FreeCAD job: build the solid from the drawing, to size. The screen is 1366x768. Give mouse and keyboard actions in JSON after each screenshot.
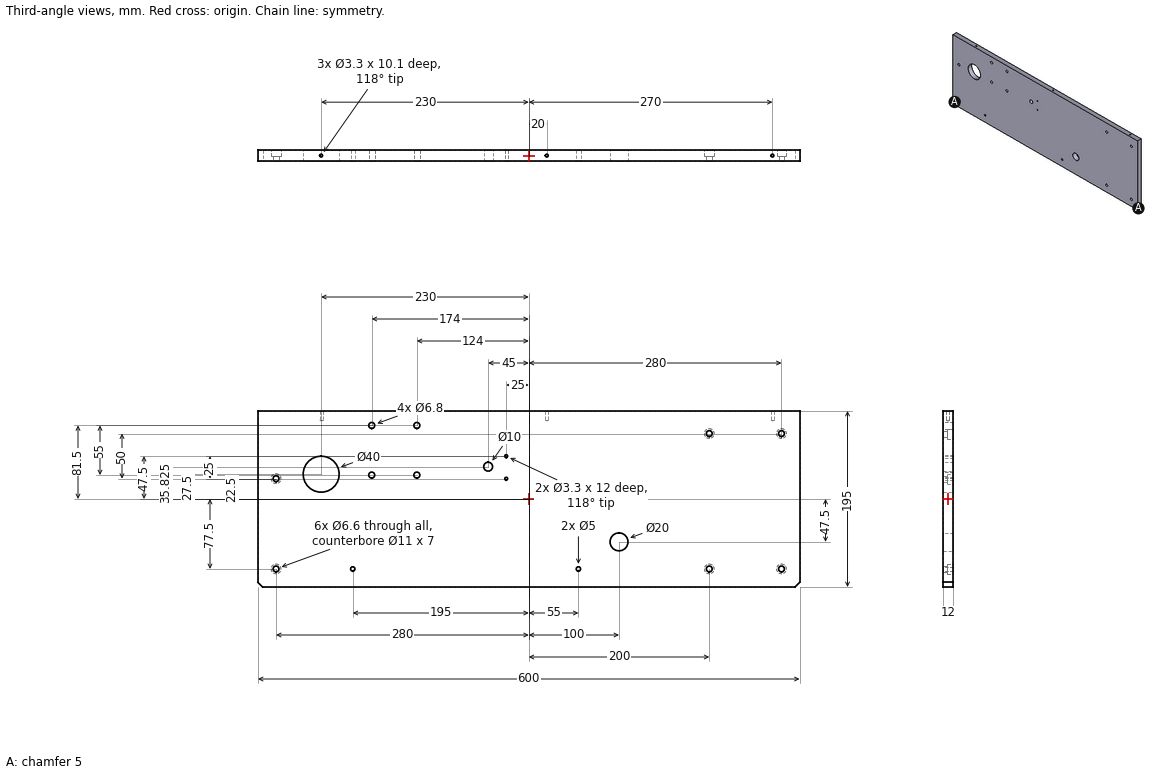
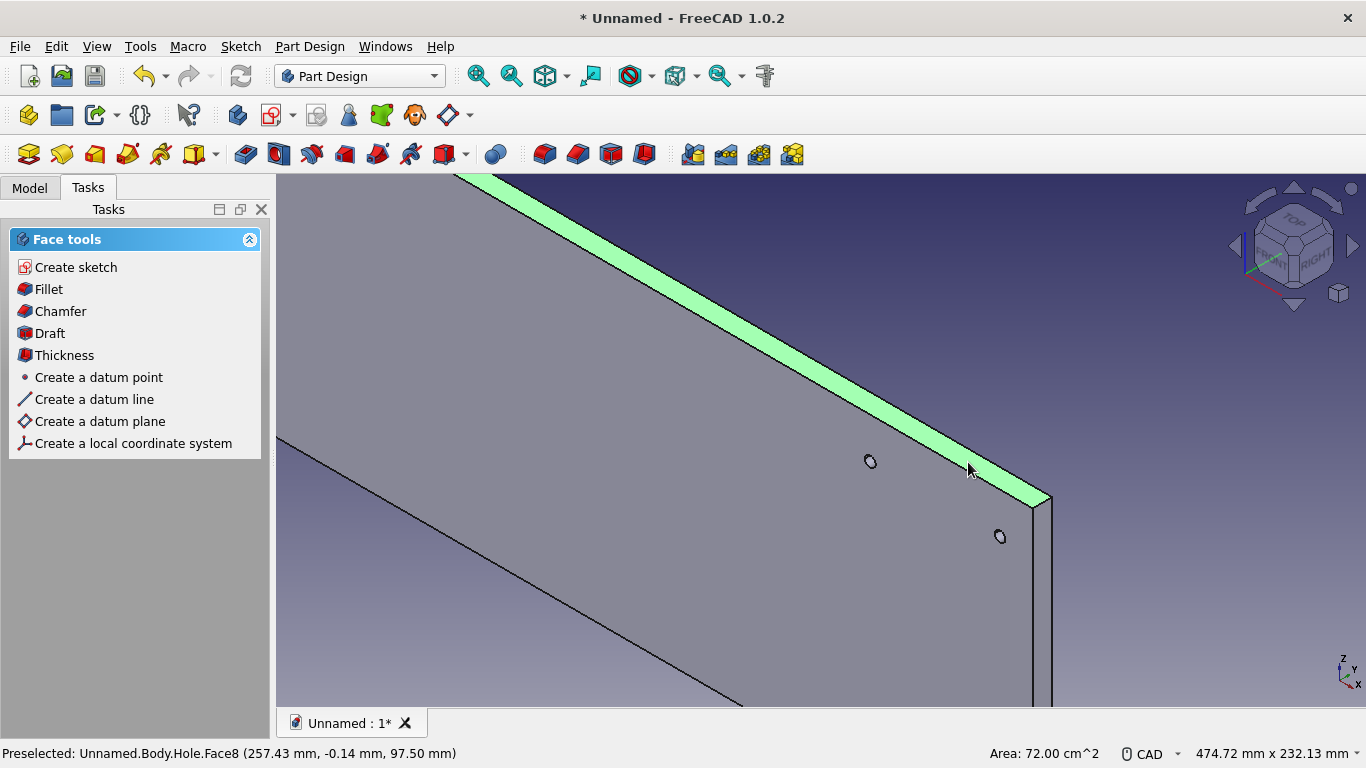
{"action": "left_click", "coordinate": [270, 116]}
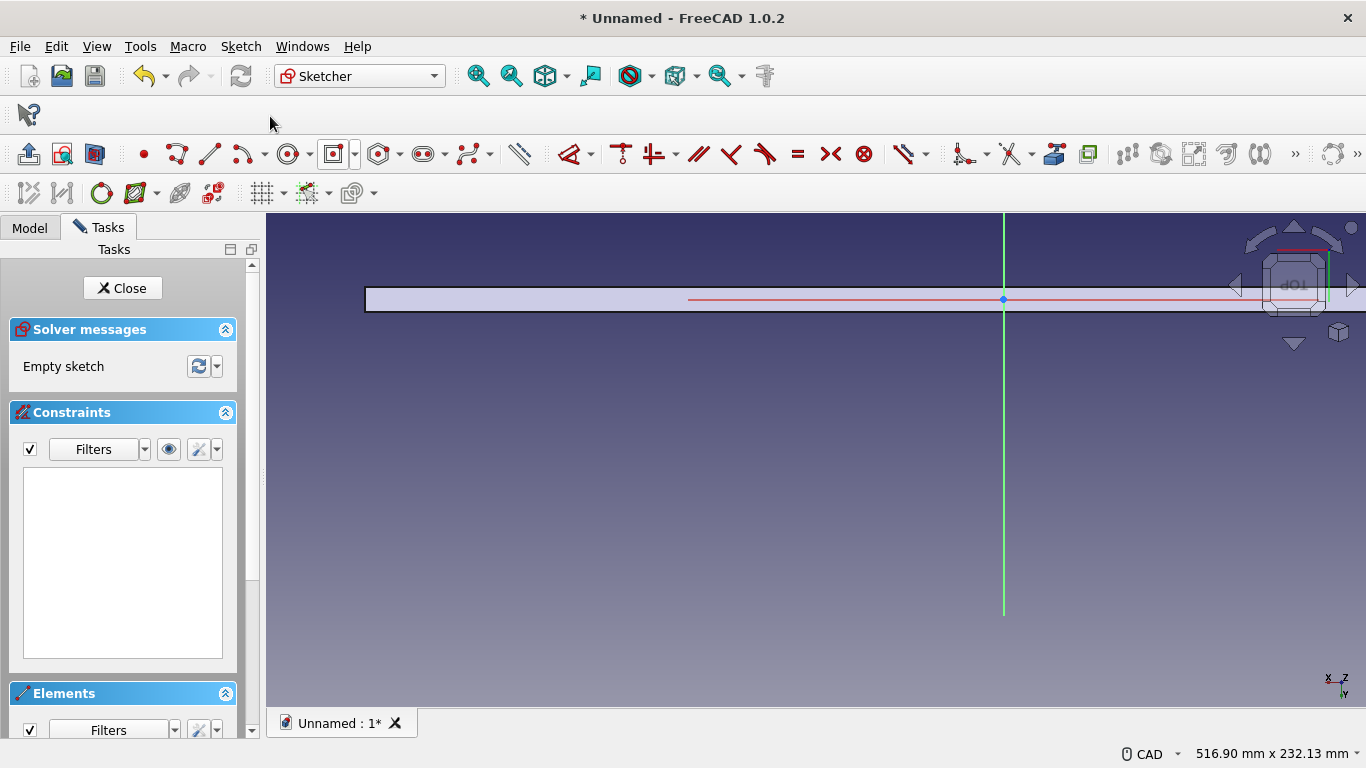
{"action": "scroll", "coordinate": [487, 655], "scroll_direction": "down", "scroll_amount": 3}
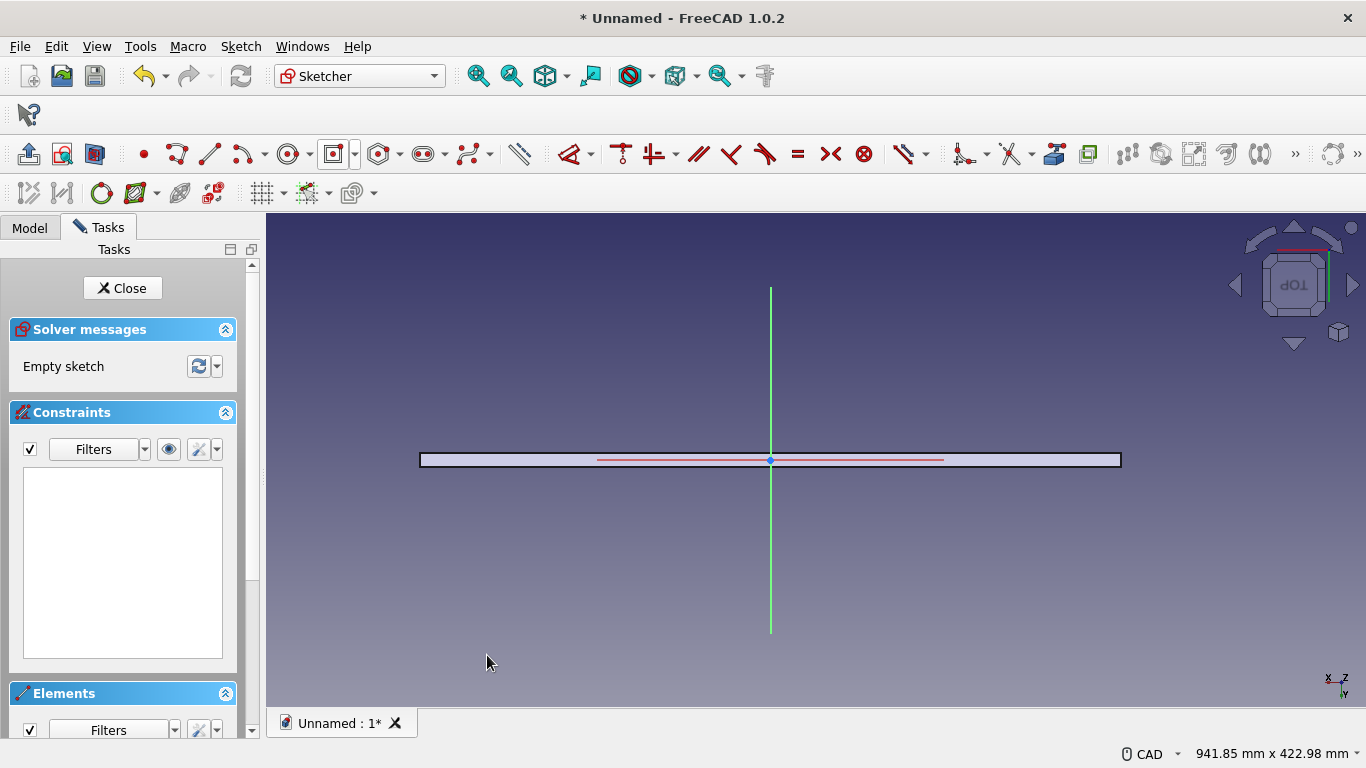
{"action": "left_click", "coordinate": [288, 154]}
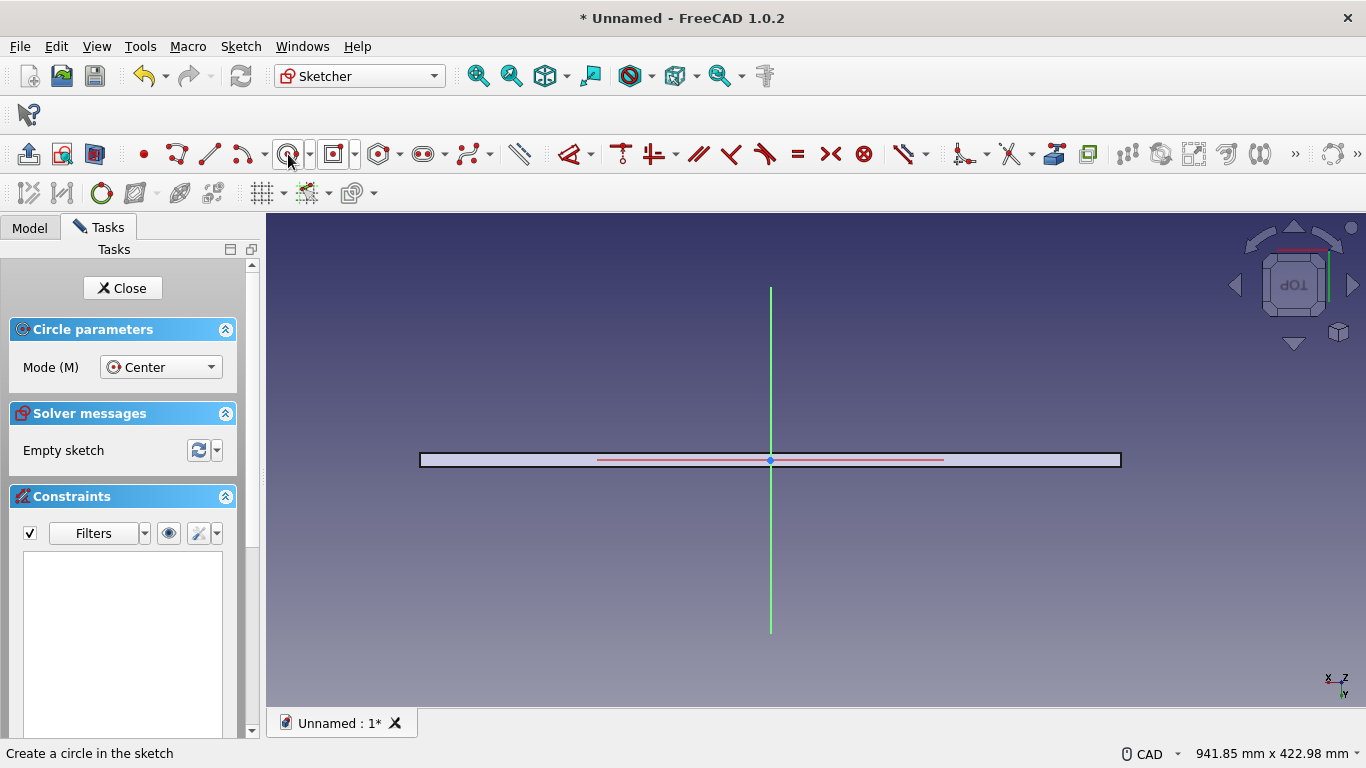
{"action": "scroll", "coordinate": [1039, 460], "scroll_direction": "up", "scroll_amount": 13}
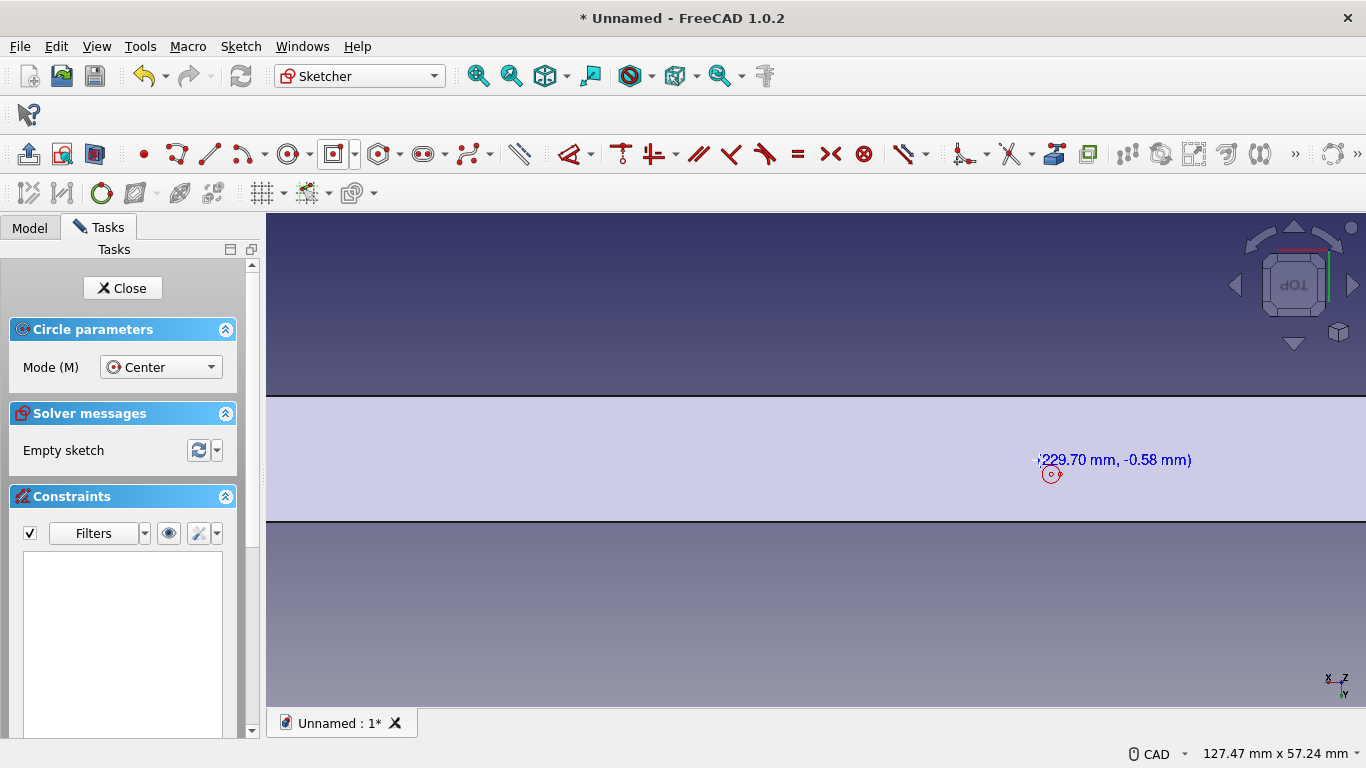
{"action": "scroll", "coordinate": [1040, 460], "scroll_direction": "down", "scroll_amount": 13}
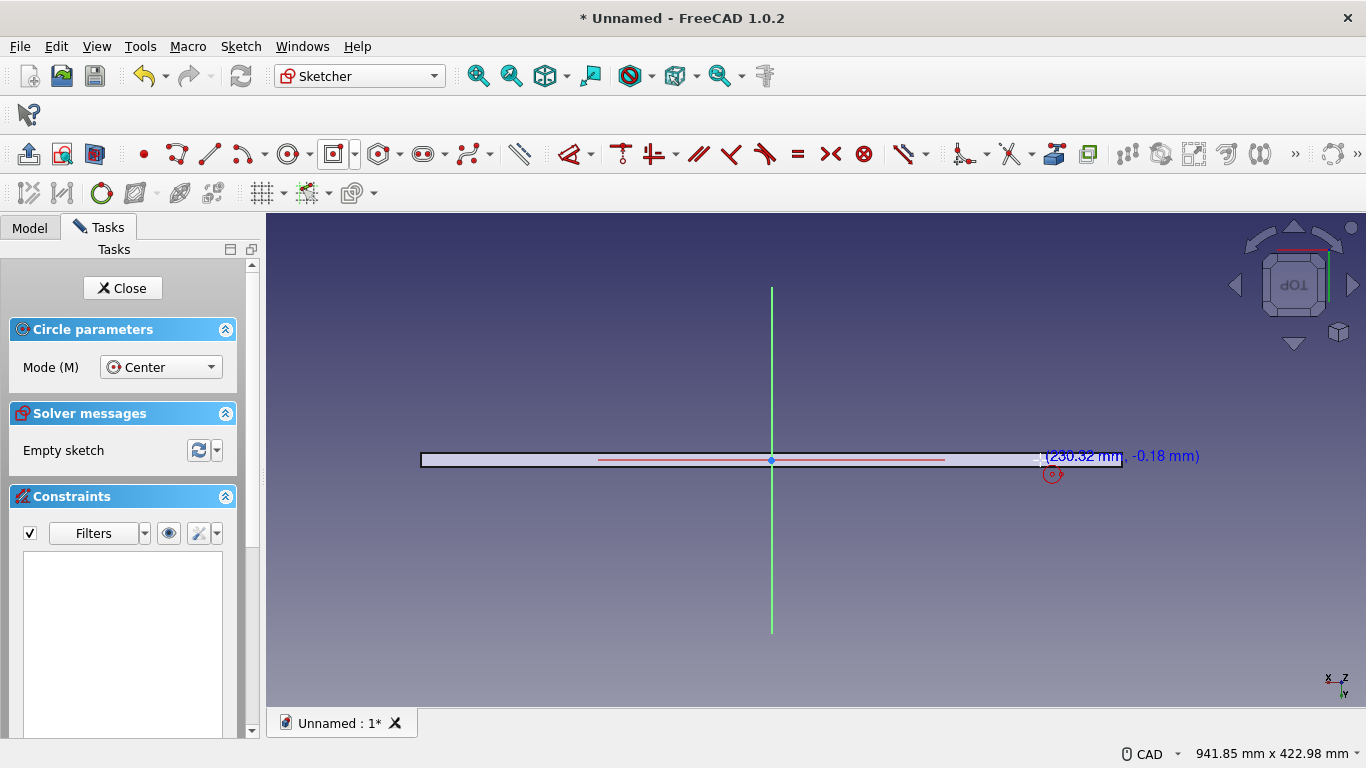
{"action": "left_click", "coordinate": [1040, 460]}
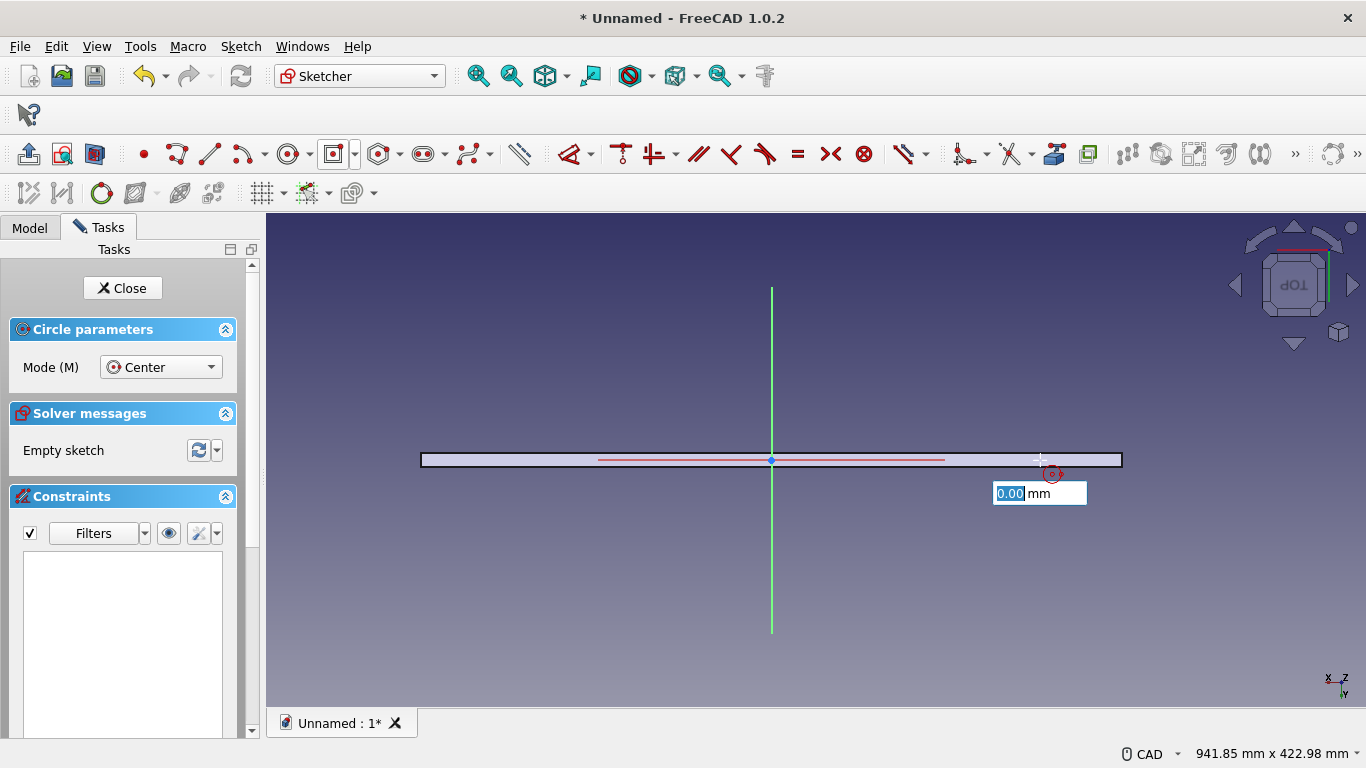
{"action": "scroll", "coordinate": [1040, 462], "scroll_direction": "up", "scroll_amount": 11}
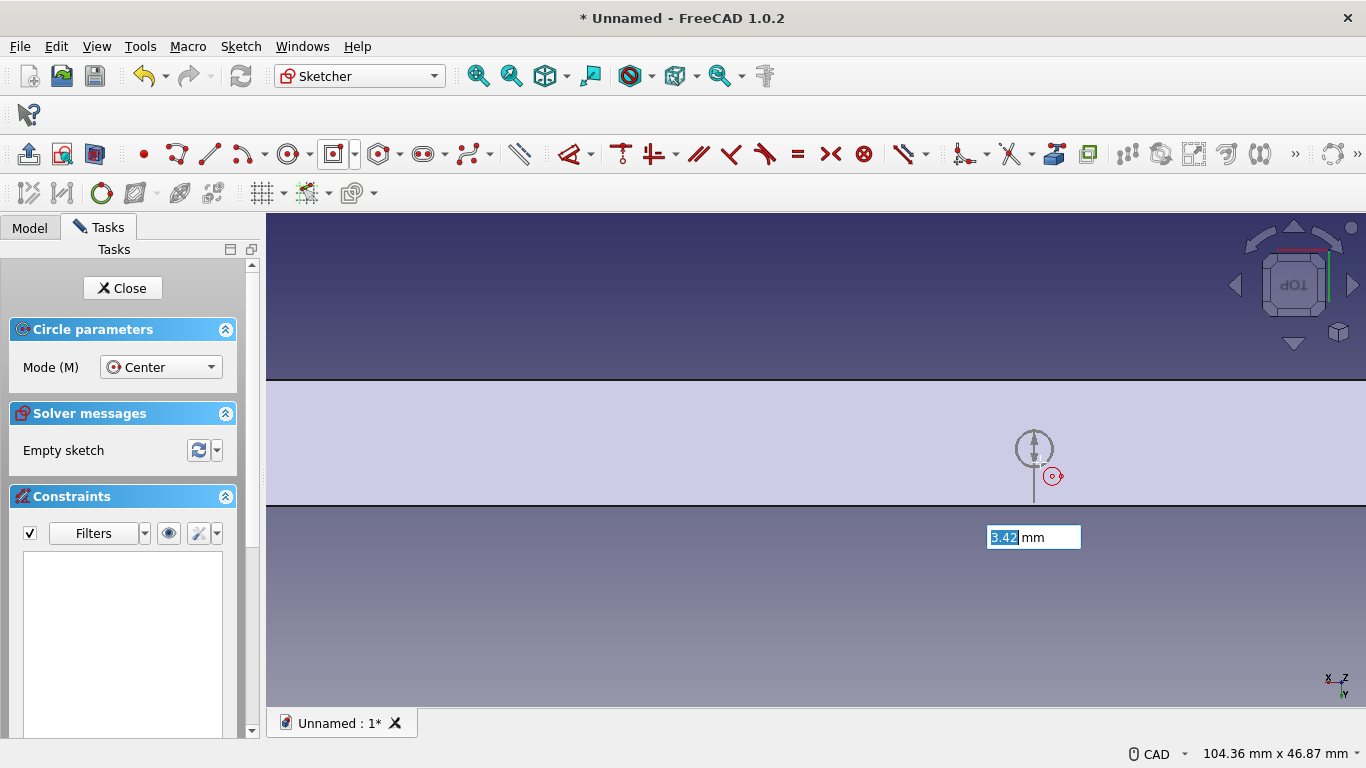
{"action": "left_click", "coordinate": [1031, 459]}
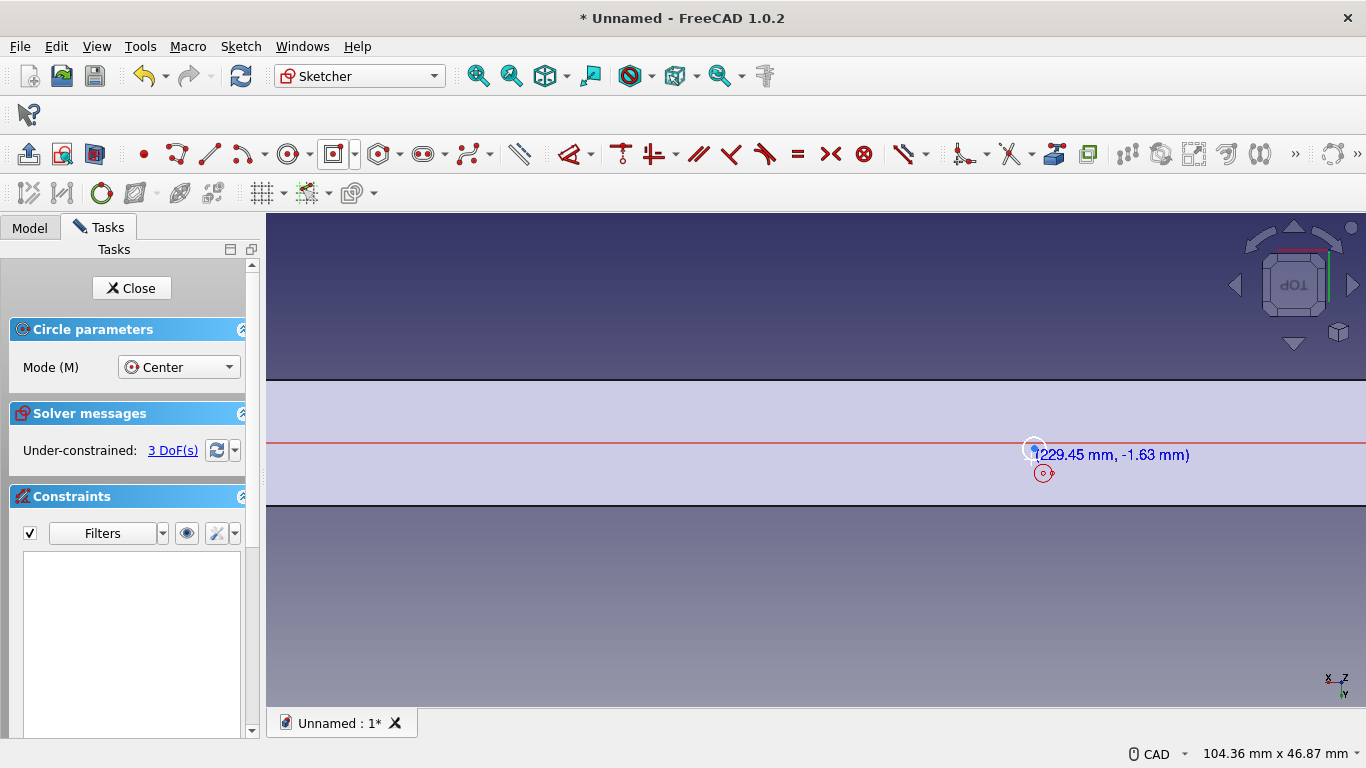
{"action": "scroll", "coordinate": [1040, 462], "scroll_direction": "down", "scroll_amount": 11}